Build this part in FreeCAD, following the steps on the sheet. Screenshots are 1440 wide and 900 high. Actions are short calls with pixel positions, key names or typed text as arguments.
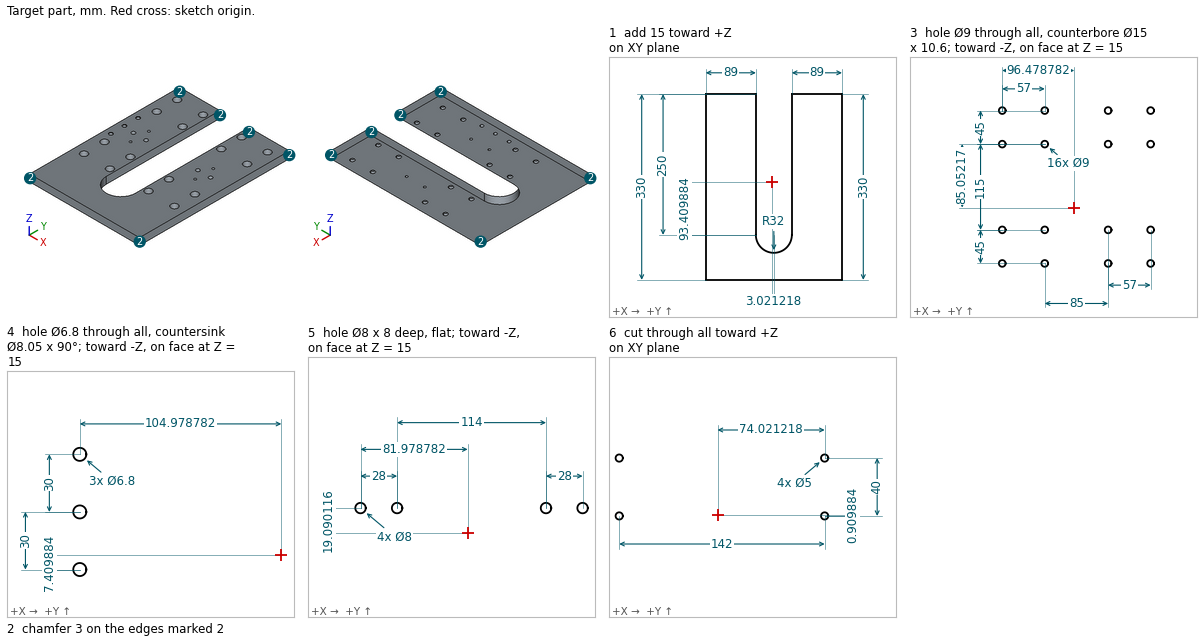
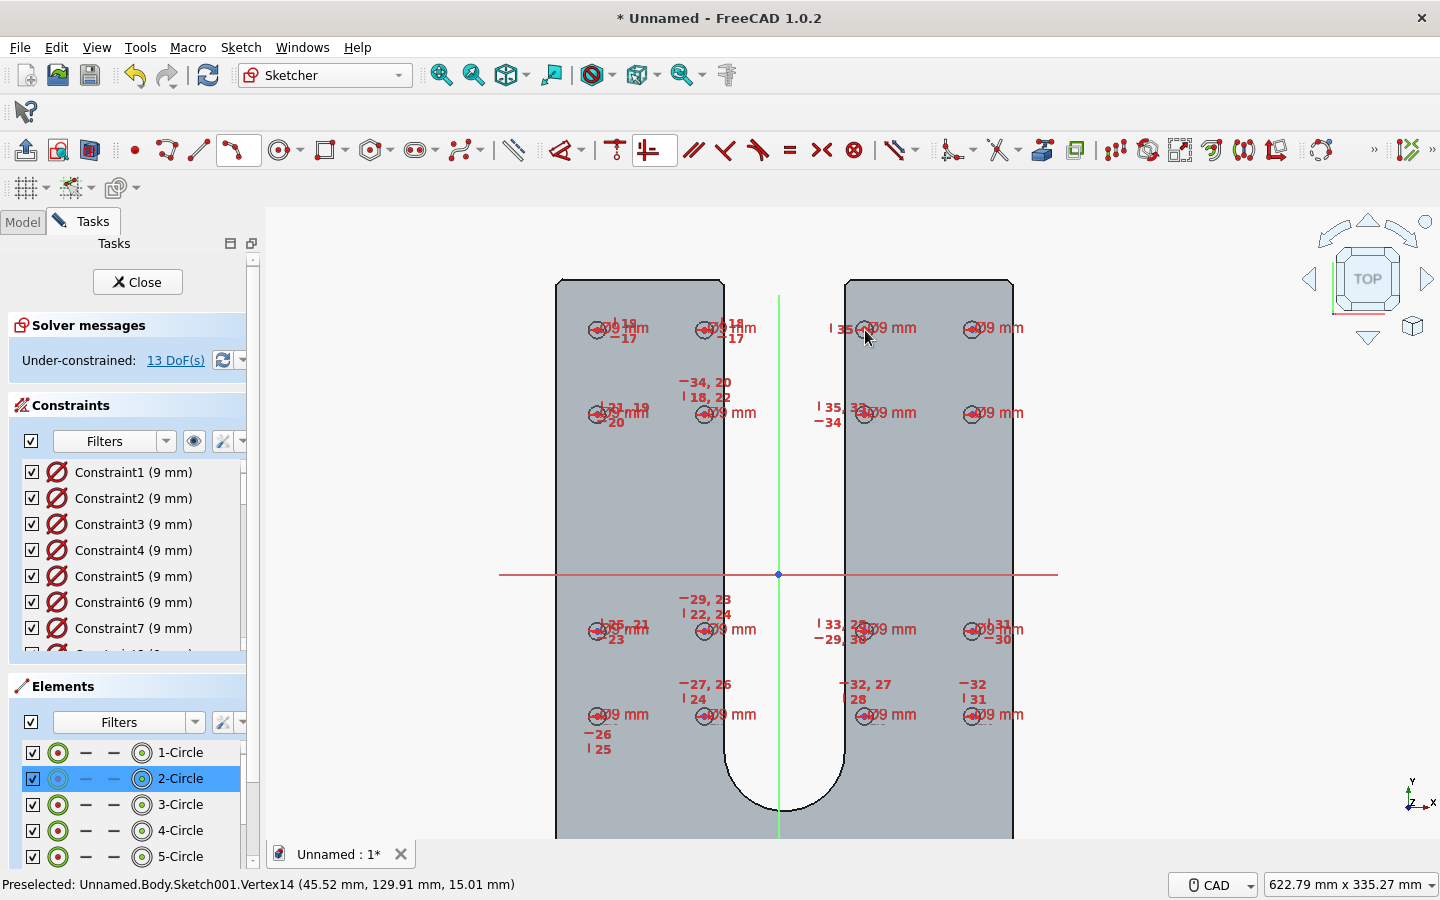
key(h)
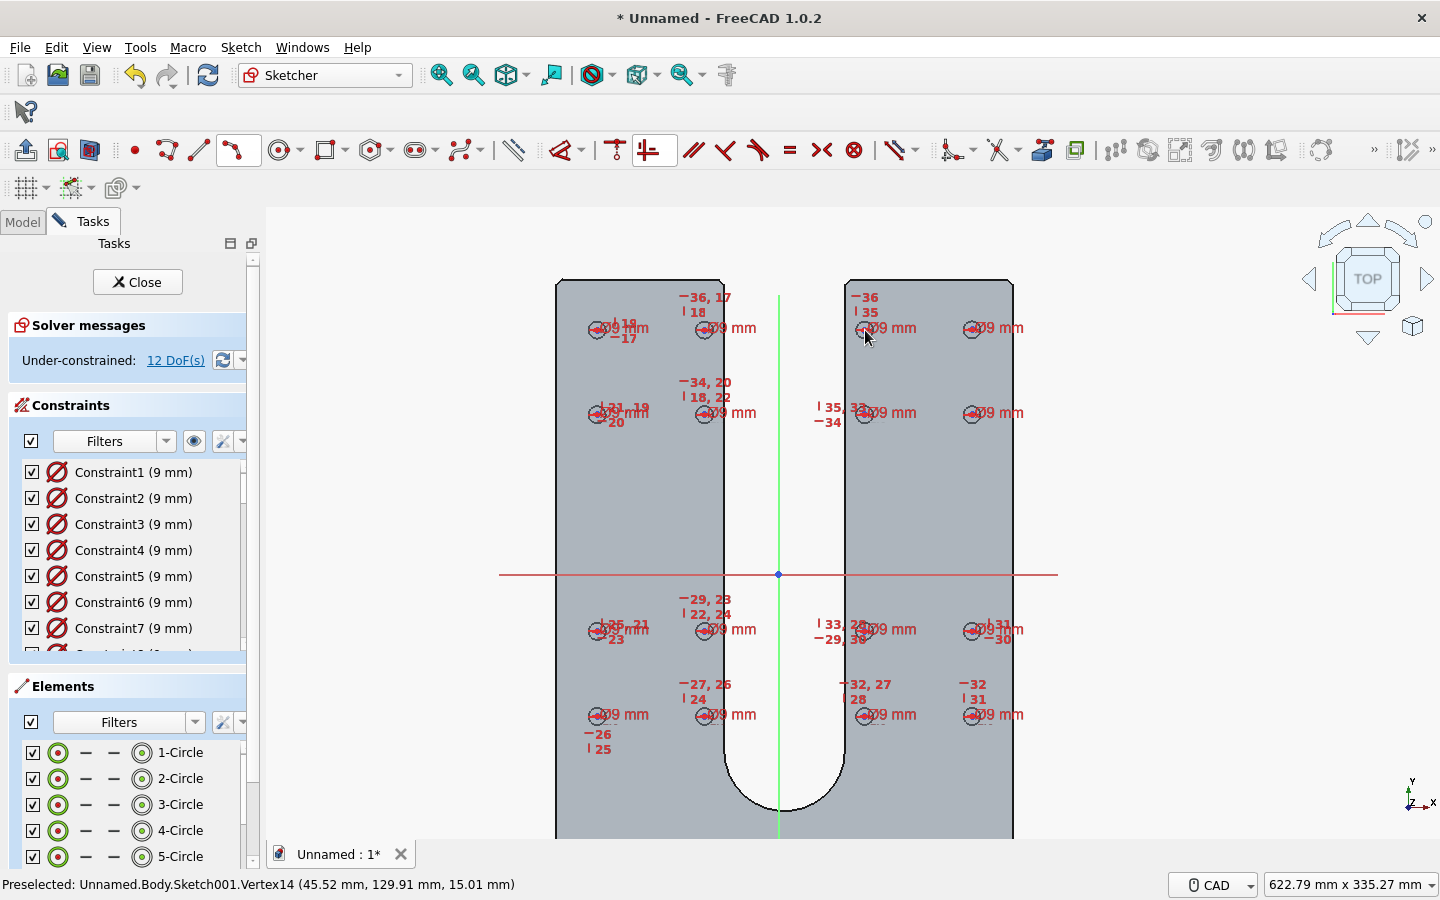
click(972, 631)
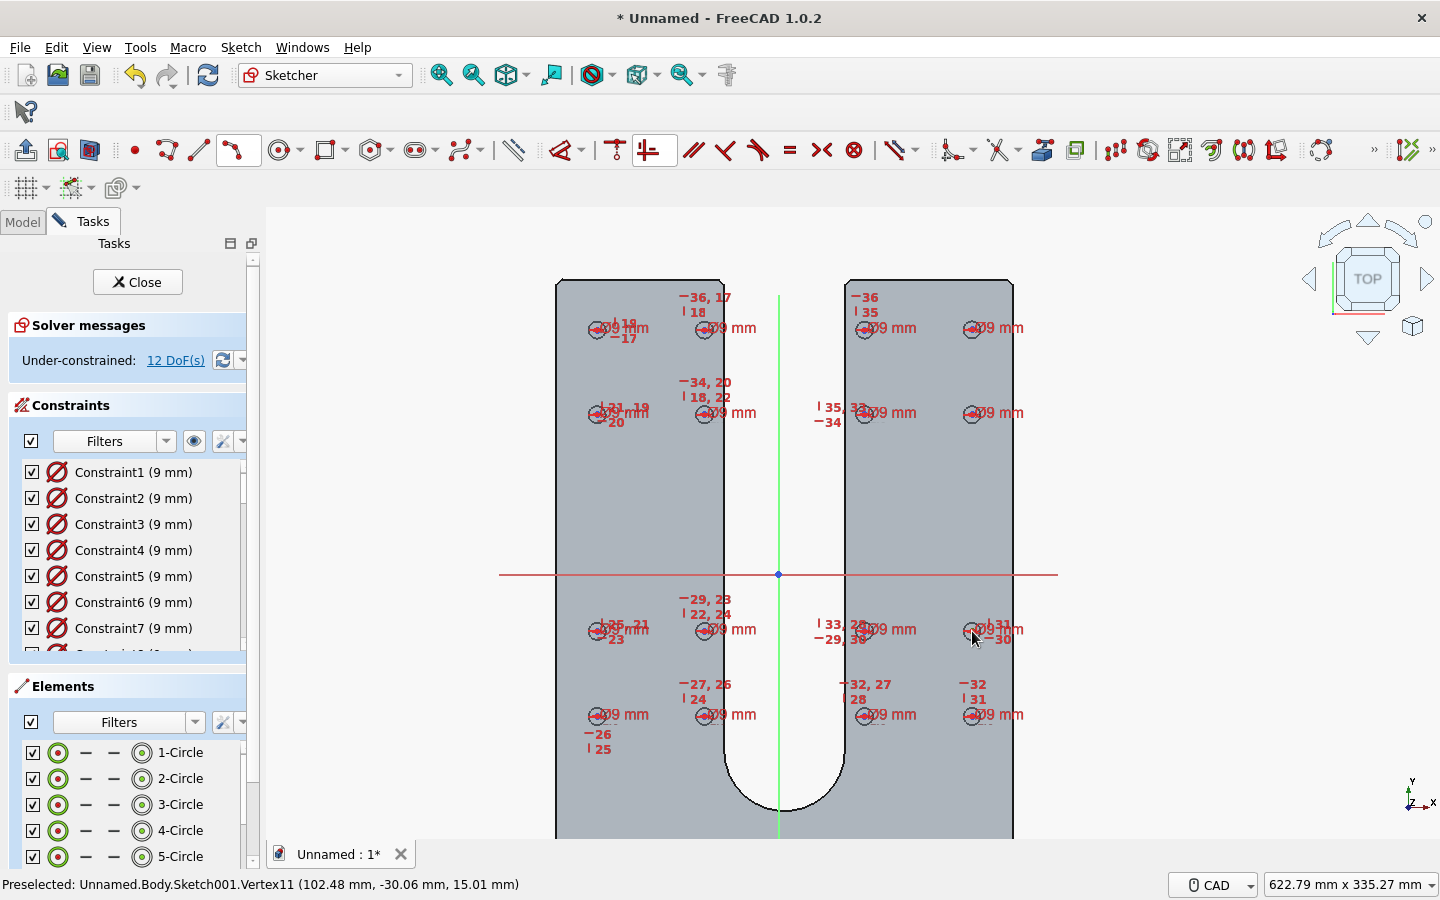
click(972, 330)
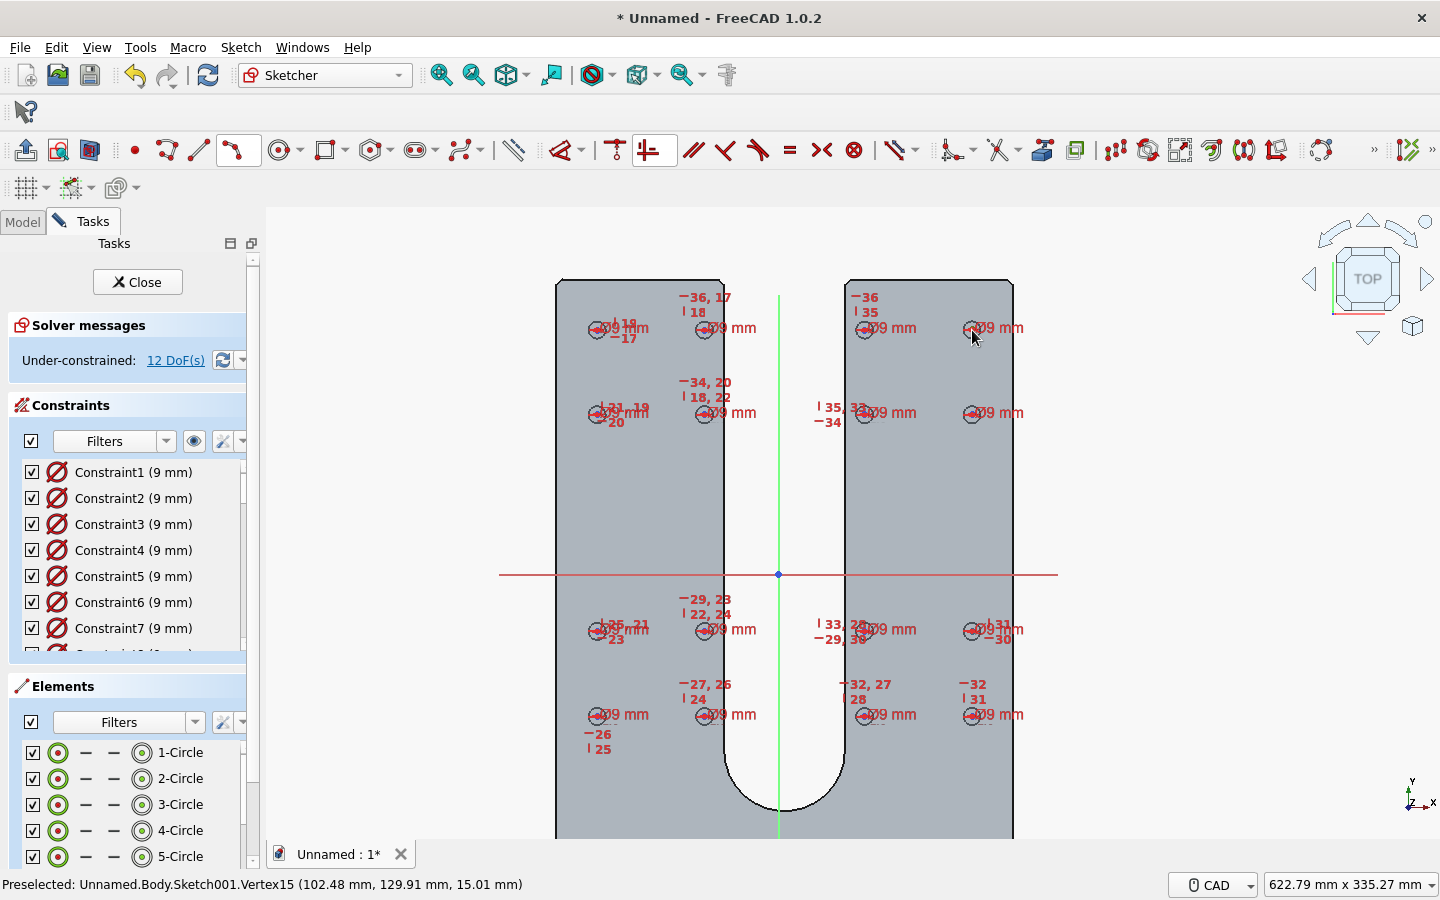
key(v)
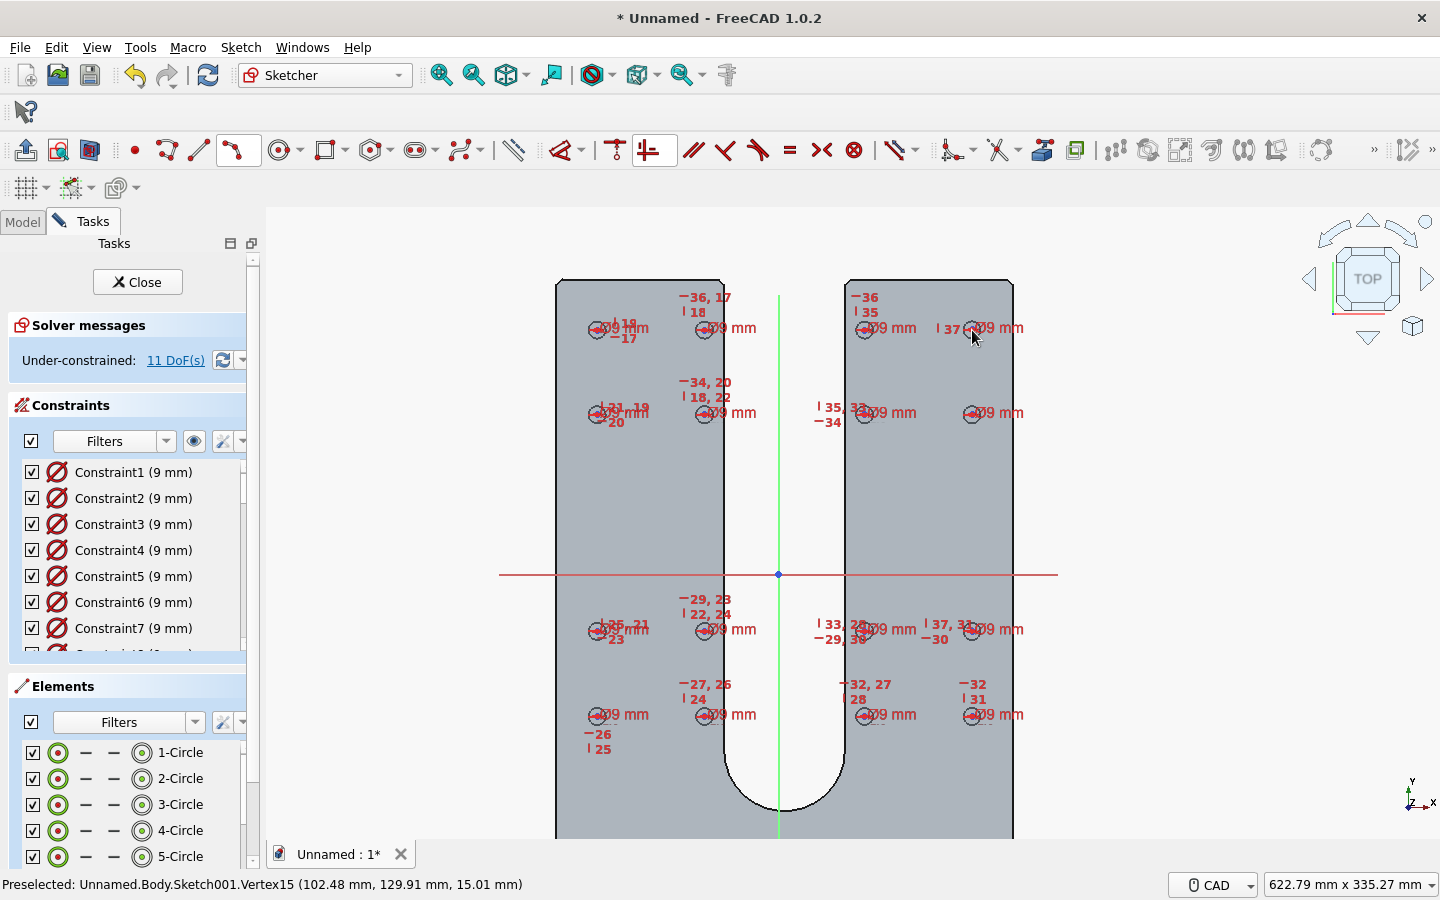
click(865, 330)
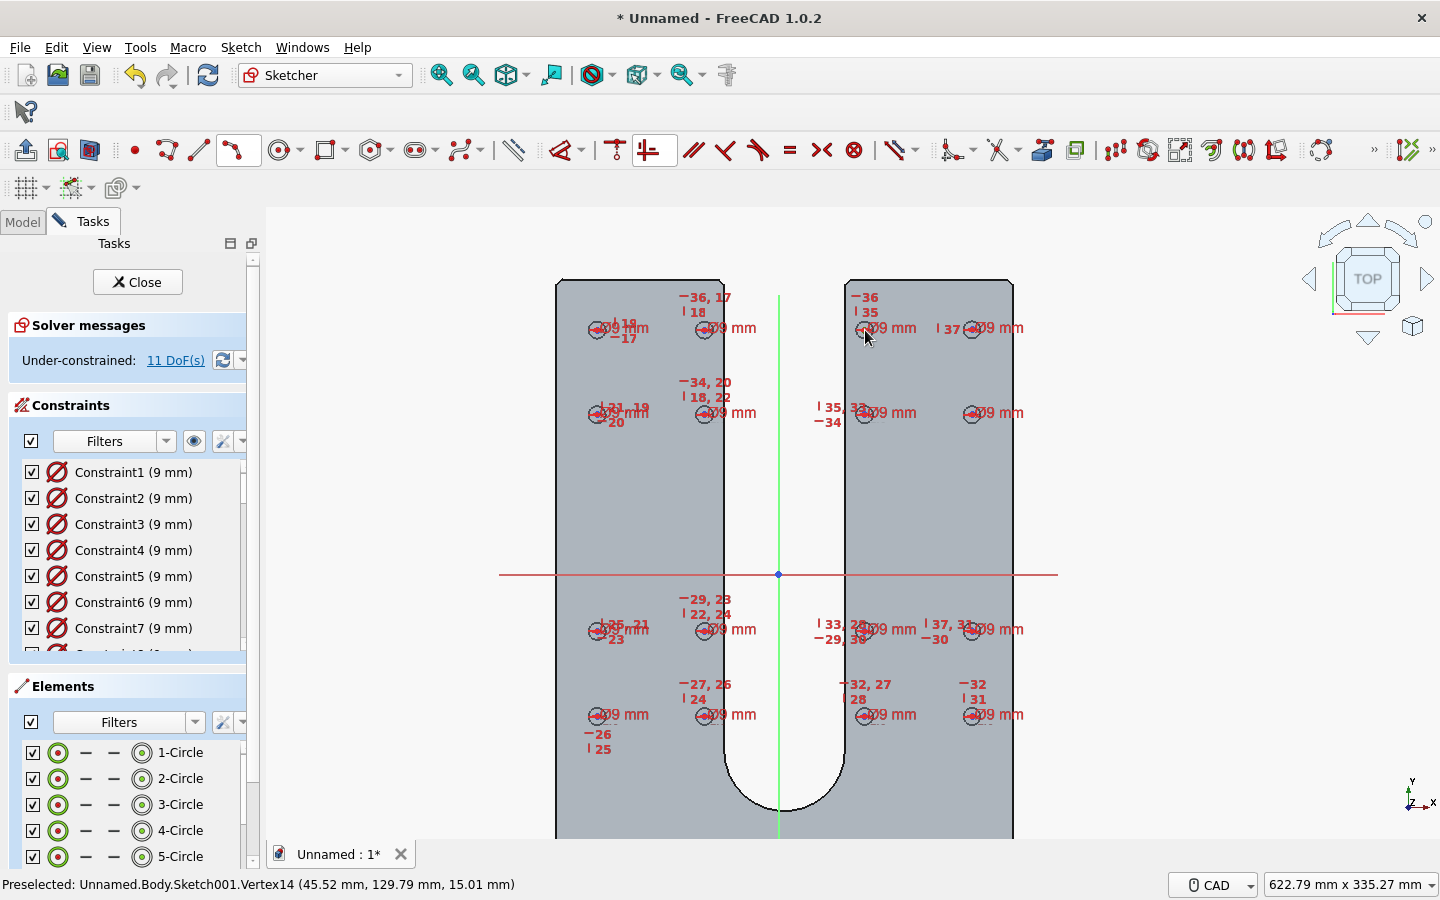
click(972, 330)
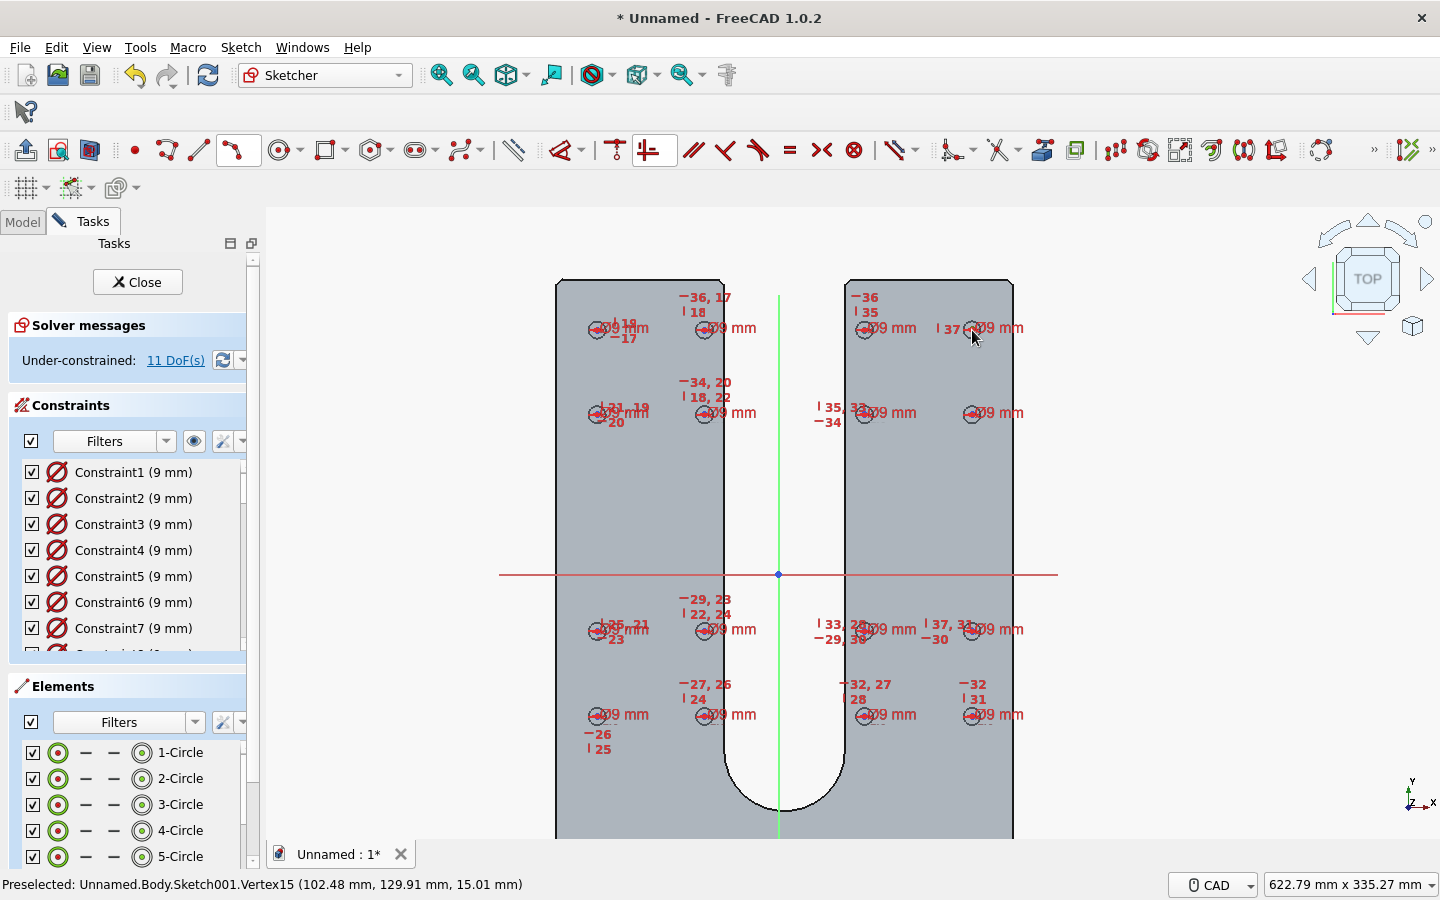
key(h)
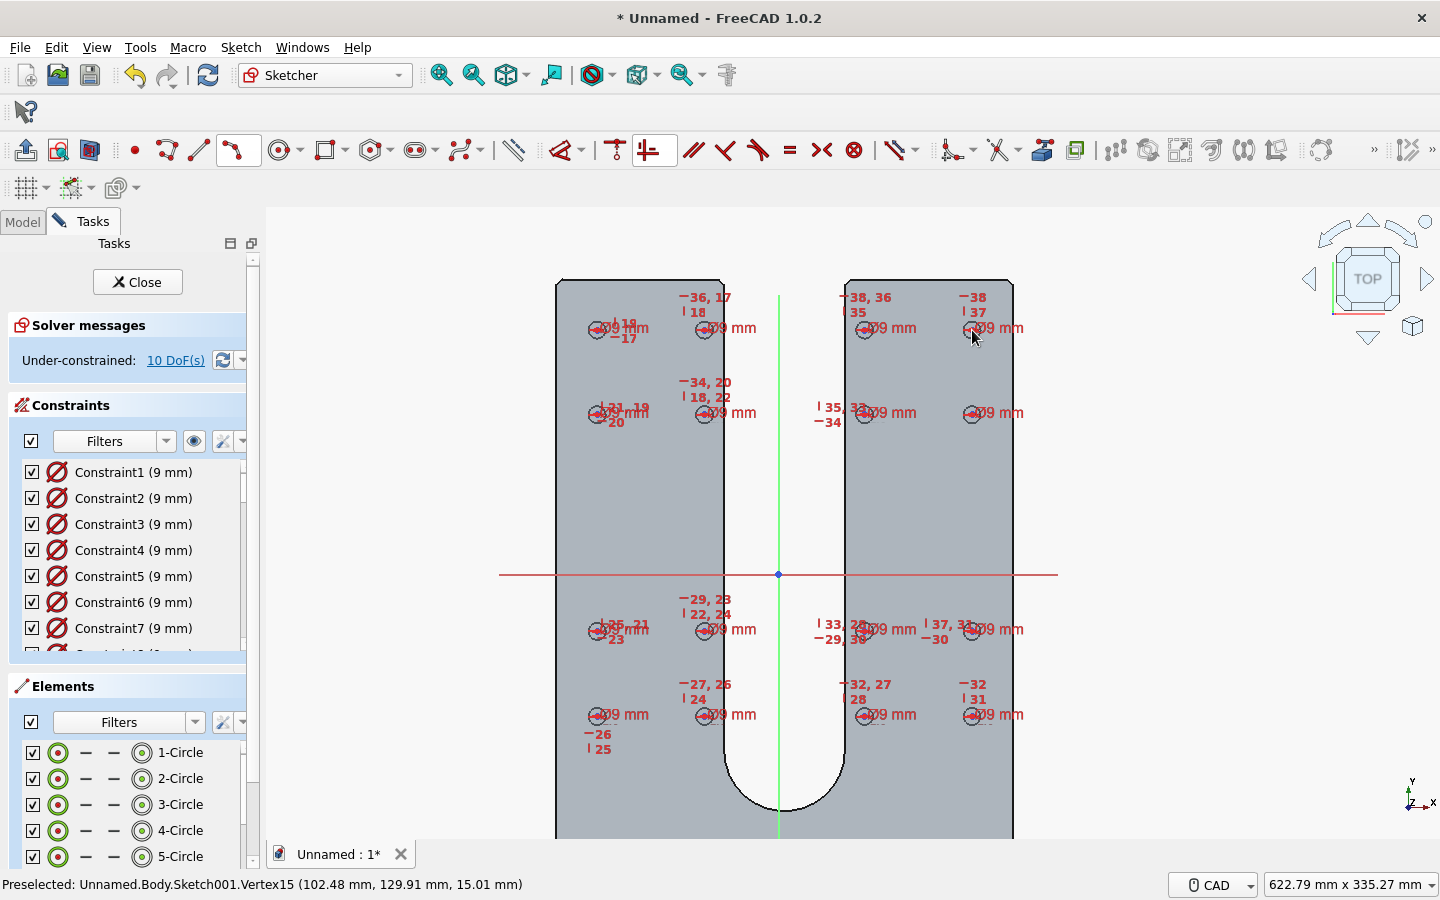
click(972, 330)